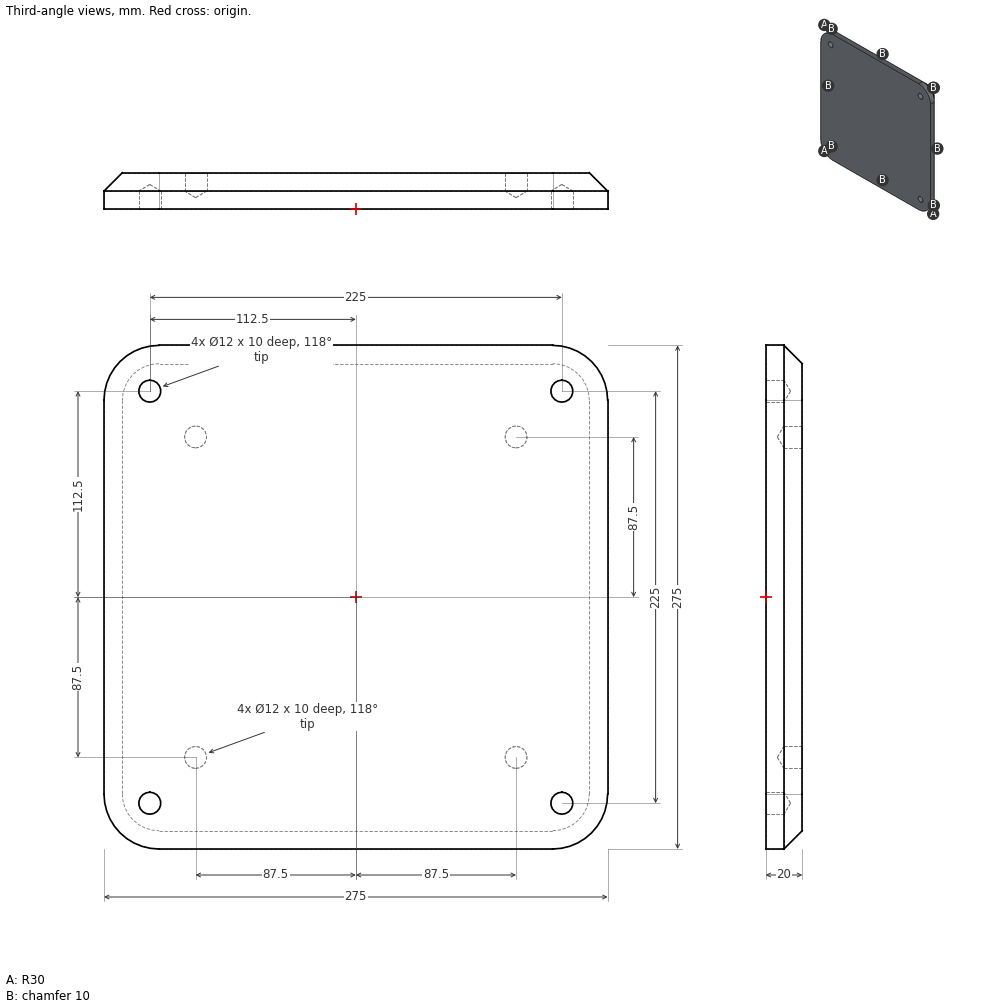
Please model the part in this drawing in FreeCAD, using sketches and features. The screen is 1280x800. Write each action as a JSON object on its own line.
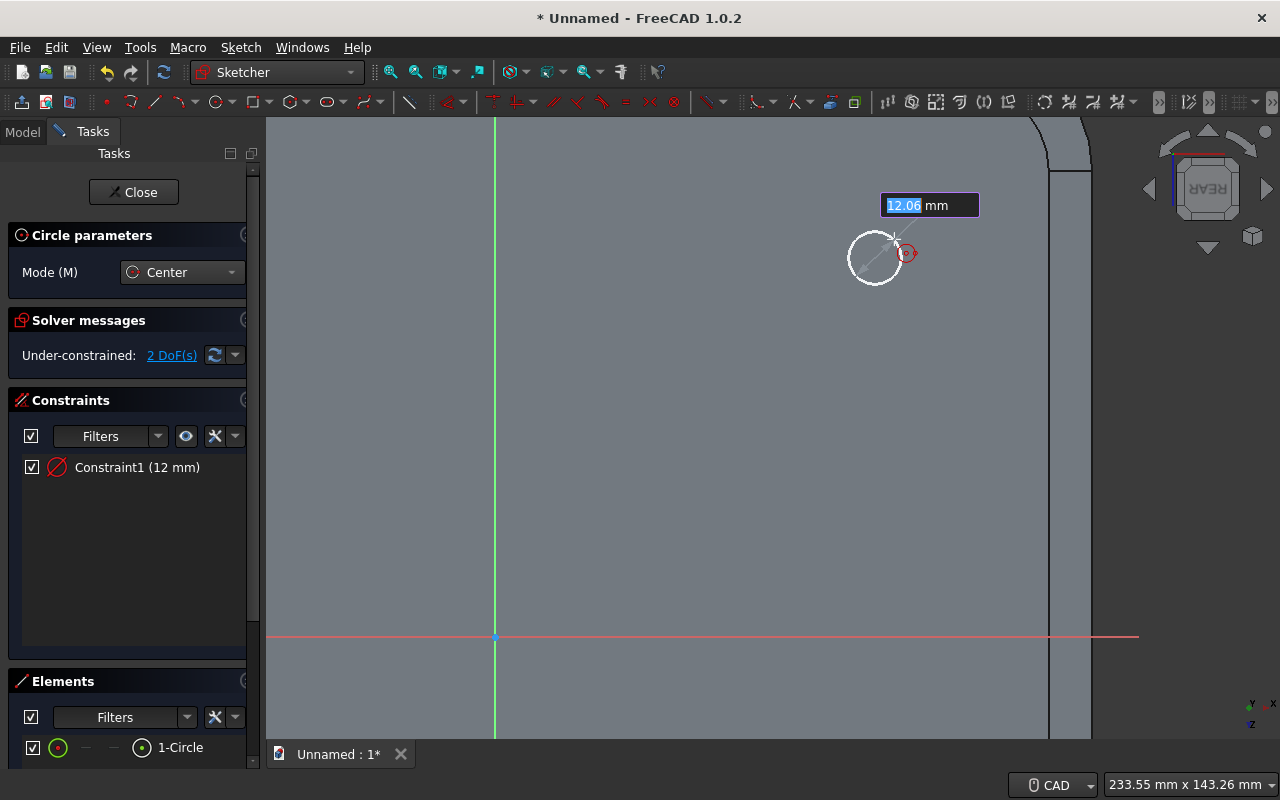
{"action": "type", "text": "12"}
{"action": "key", "text": "Return"}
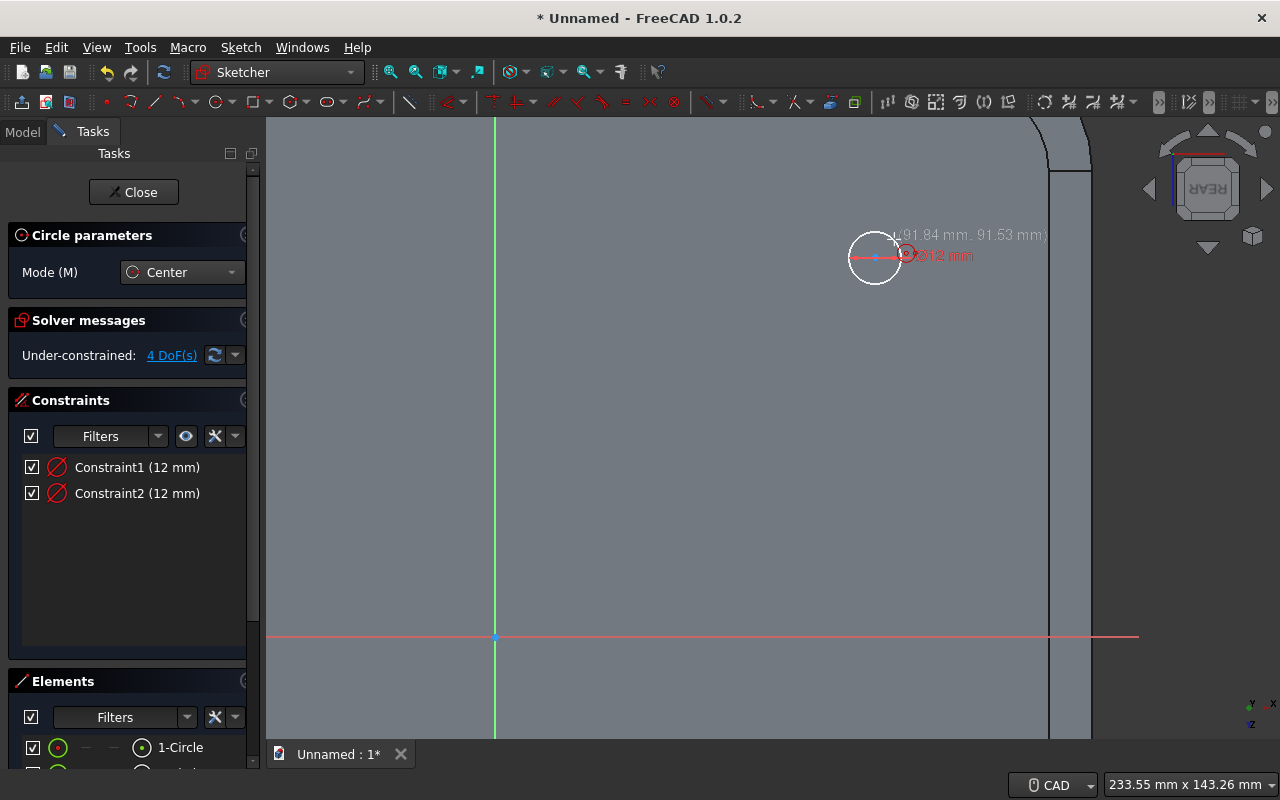
{"action": "scroll", "coordinate": [875, 257], "scroll_direction": "down", "scroll_amount": 4}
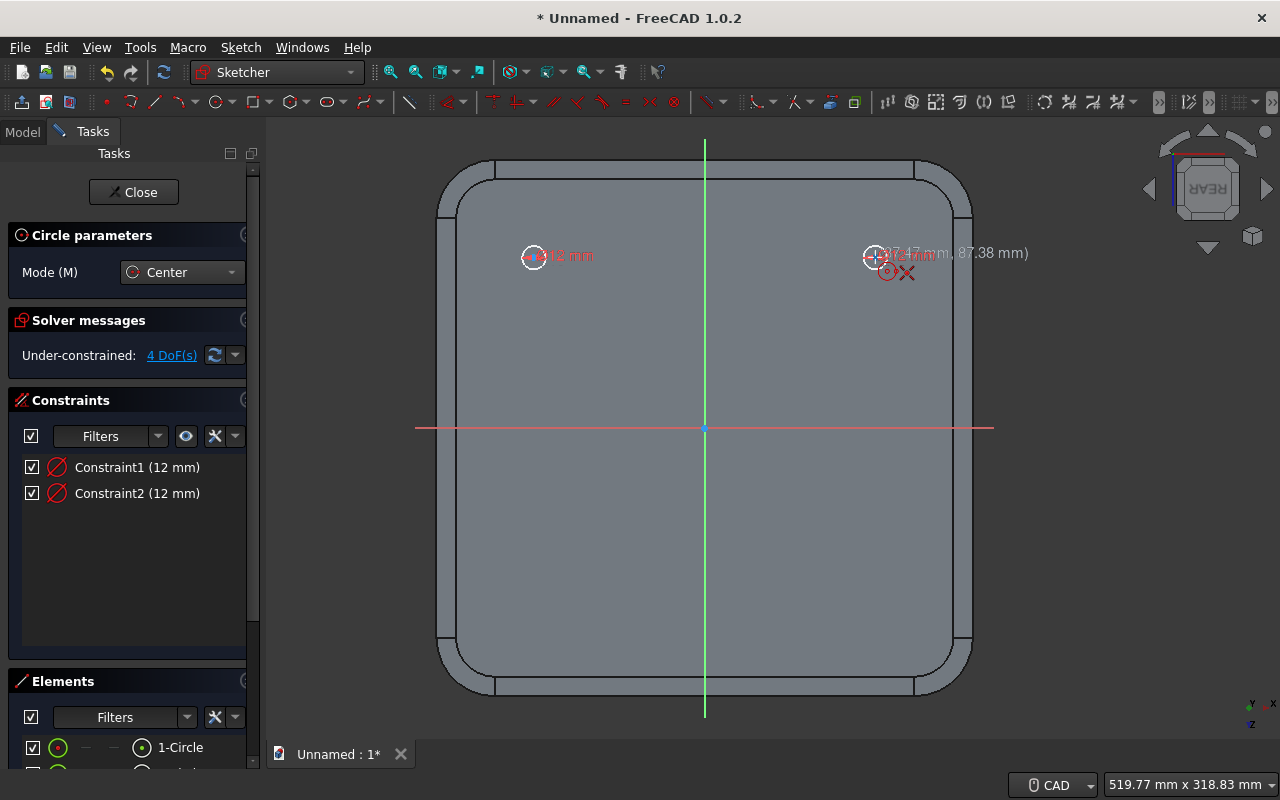
{"action": "scroll", "coordinate": [875, 599], "scroll_direction": "up", "scroll_amount": 4}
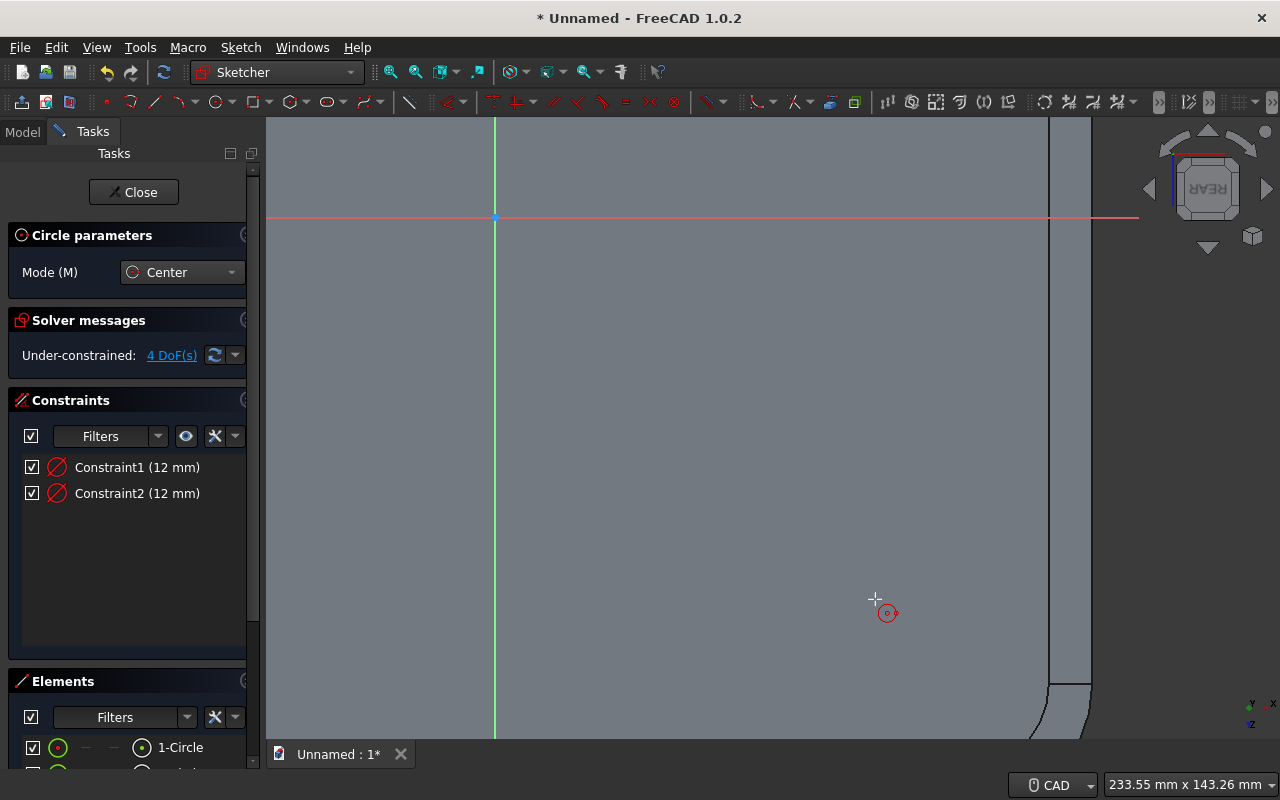
{"action": "left_click", "coordinate": [875, 597]}
{"action": "mouse_move", "coordinate": [894, 579]}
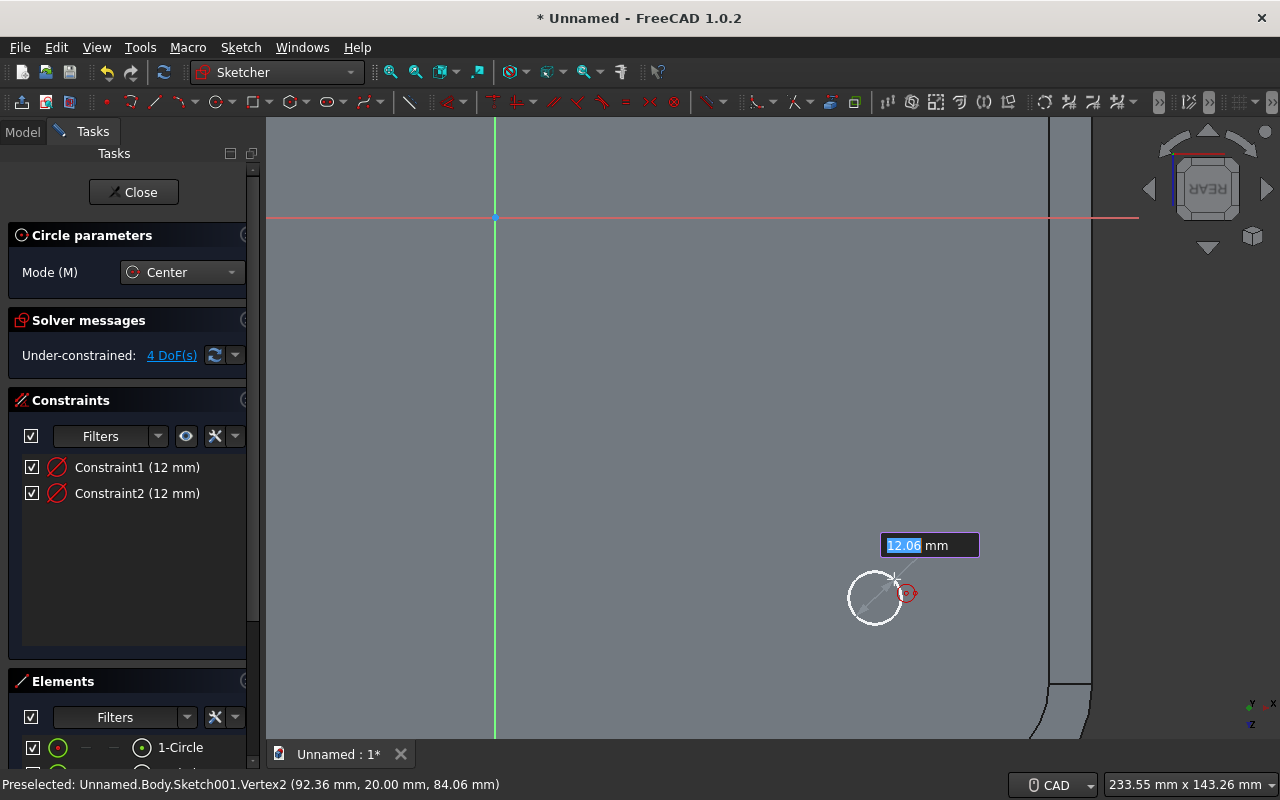
{"action": "type", "text": "12"}
{"action": "key", "text": "Return"}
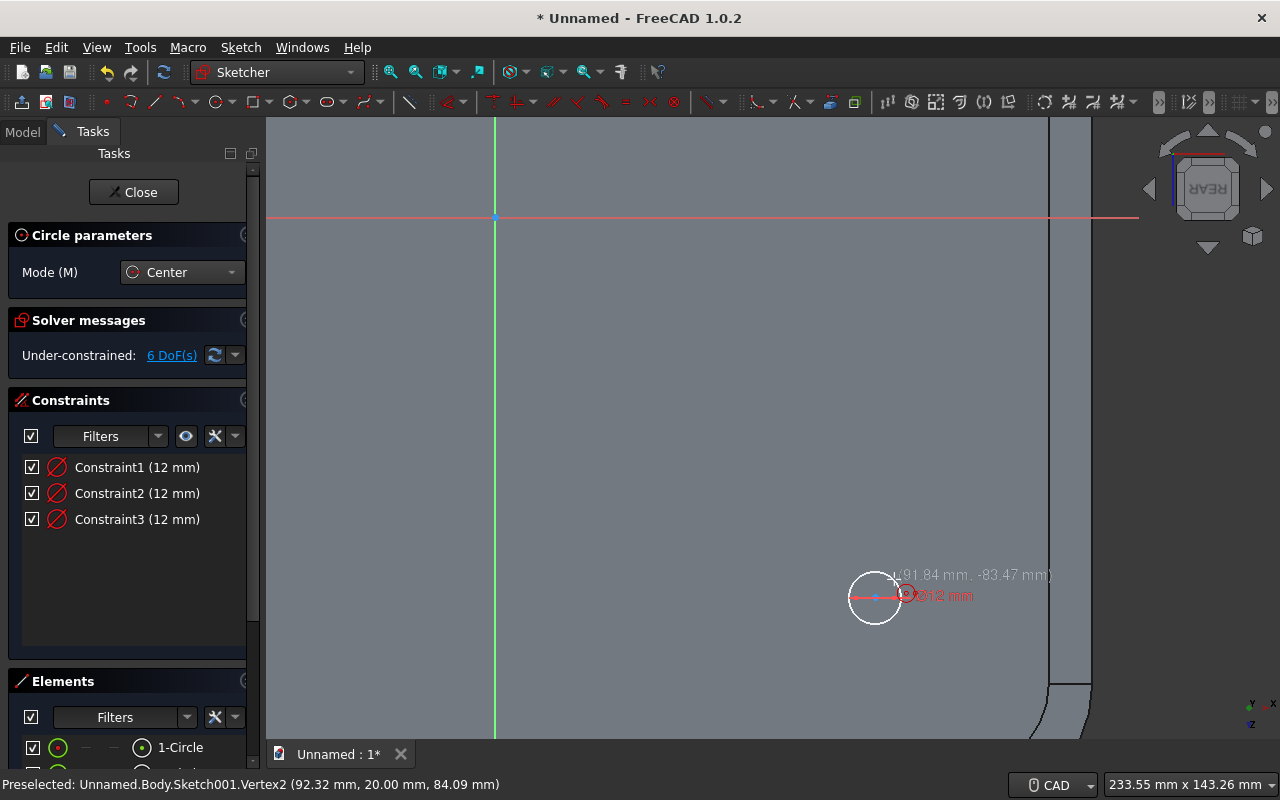
{"action": "scroll", "coordinate": [875, 600], "scroll_direction": "down", "scroll_amount": 4}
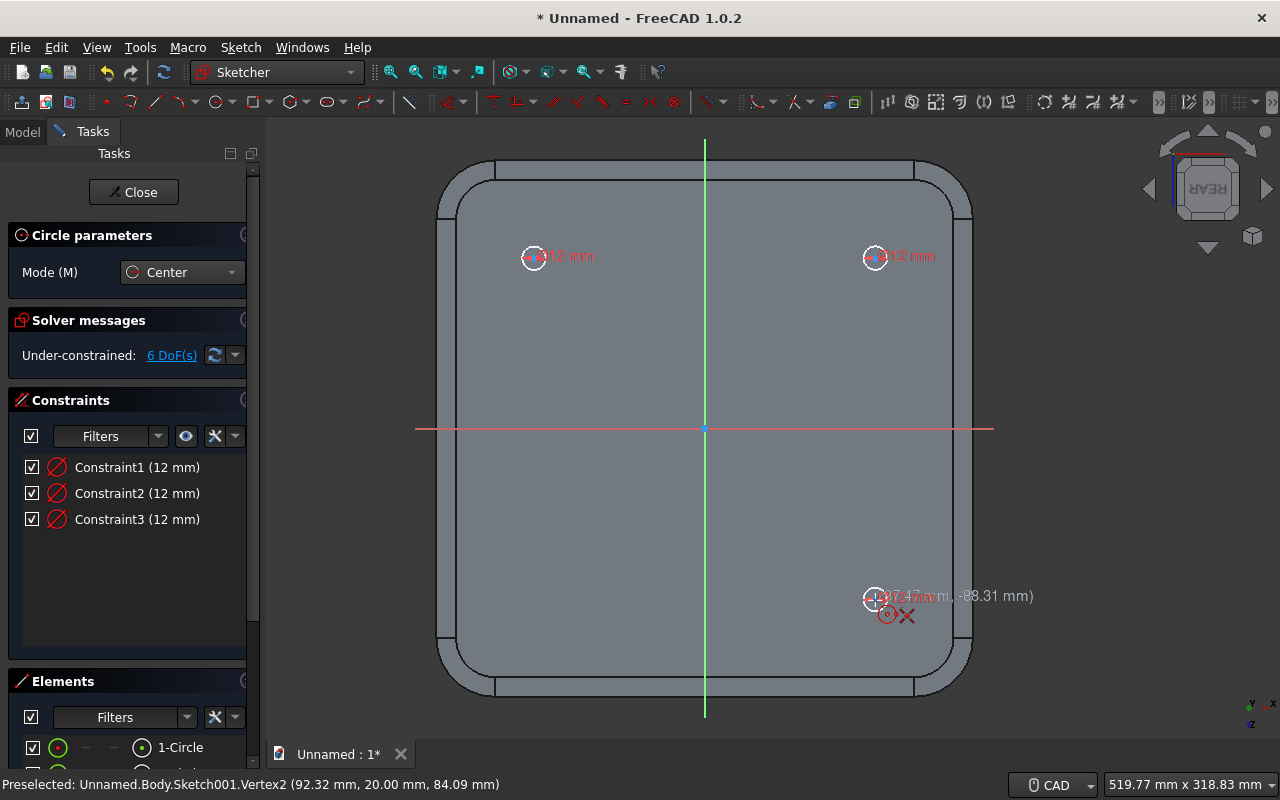
{"action": "scroll", "coordinate": [534, 599], "scroll_direction": "up", "scroll_amount": 4}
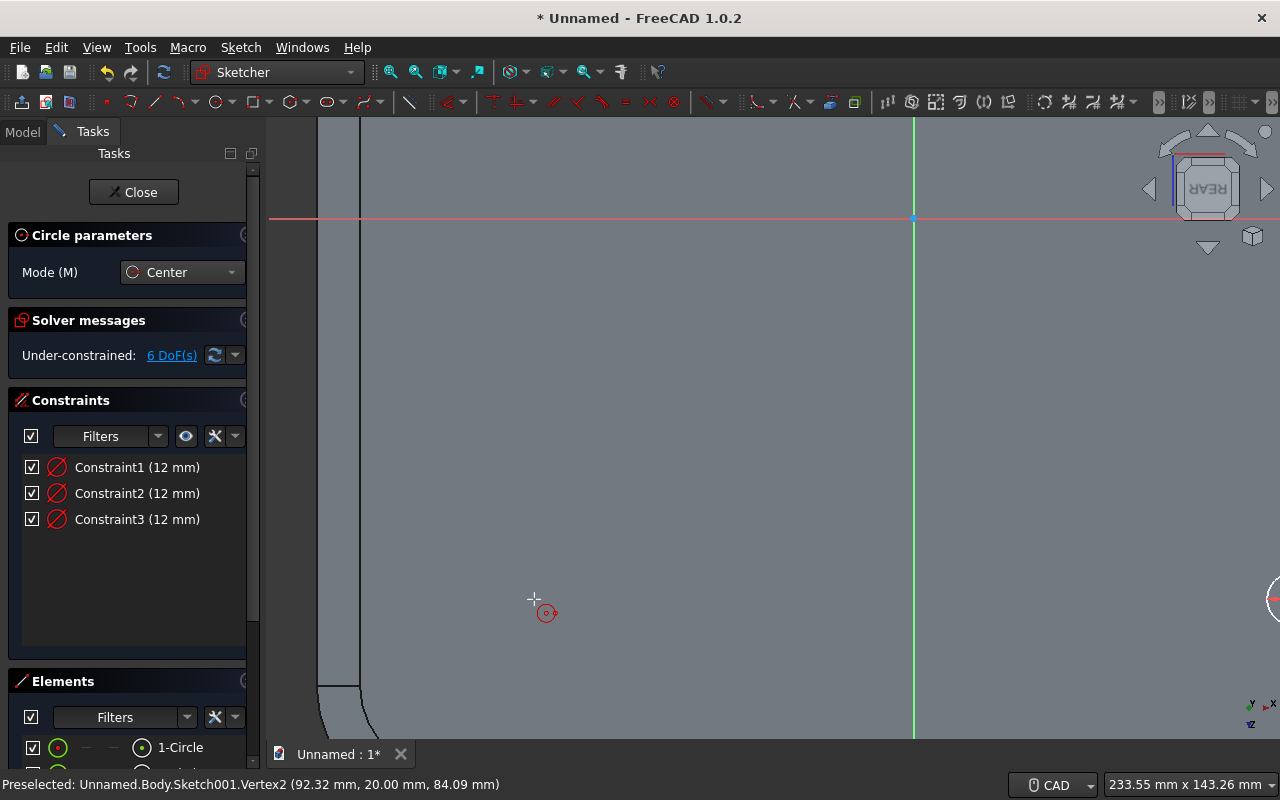
{"action": "left_click", "coordinate": [534, 599]}
{"action": "mouse_move", "coordinate": [552, 580]}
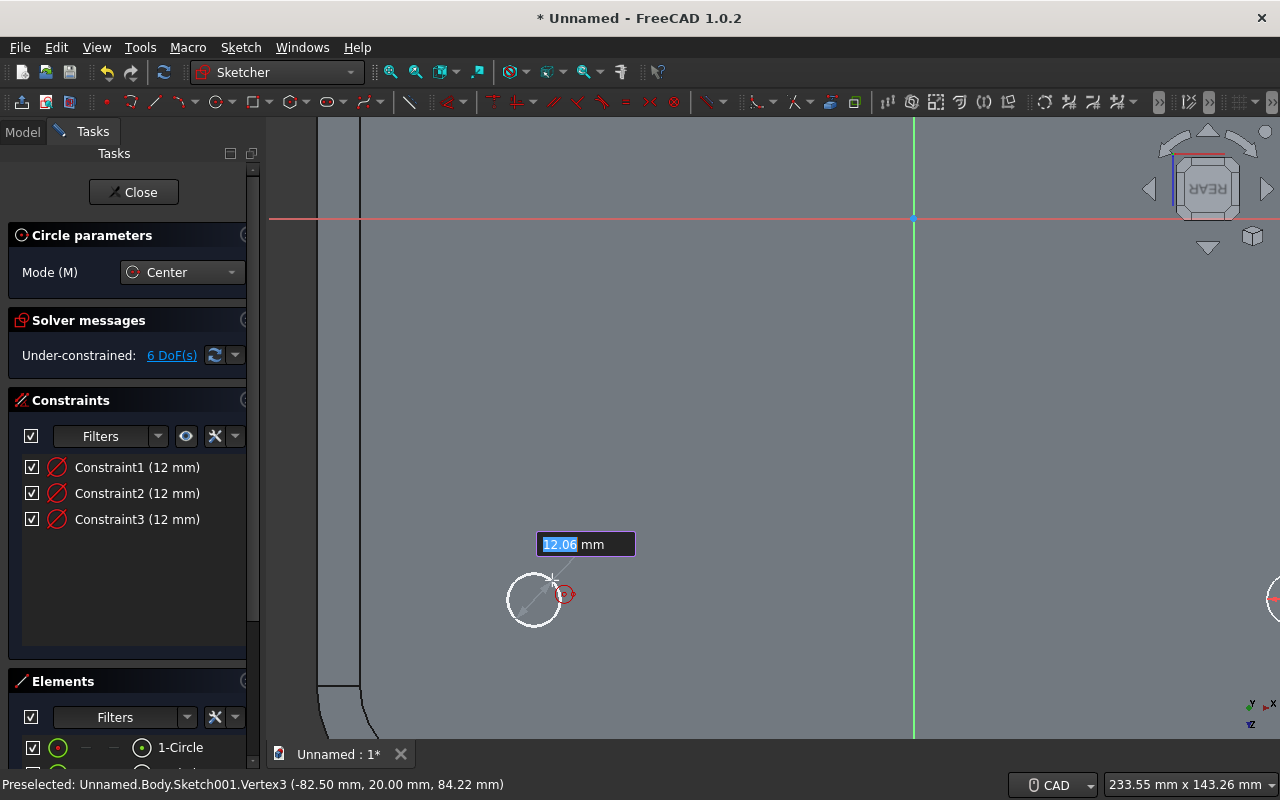
{"action": "type", "text": "12"}
{"action": "key", "text": "Return"}
{"action": "key", "text": "Escape"}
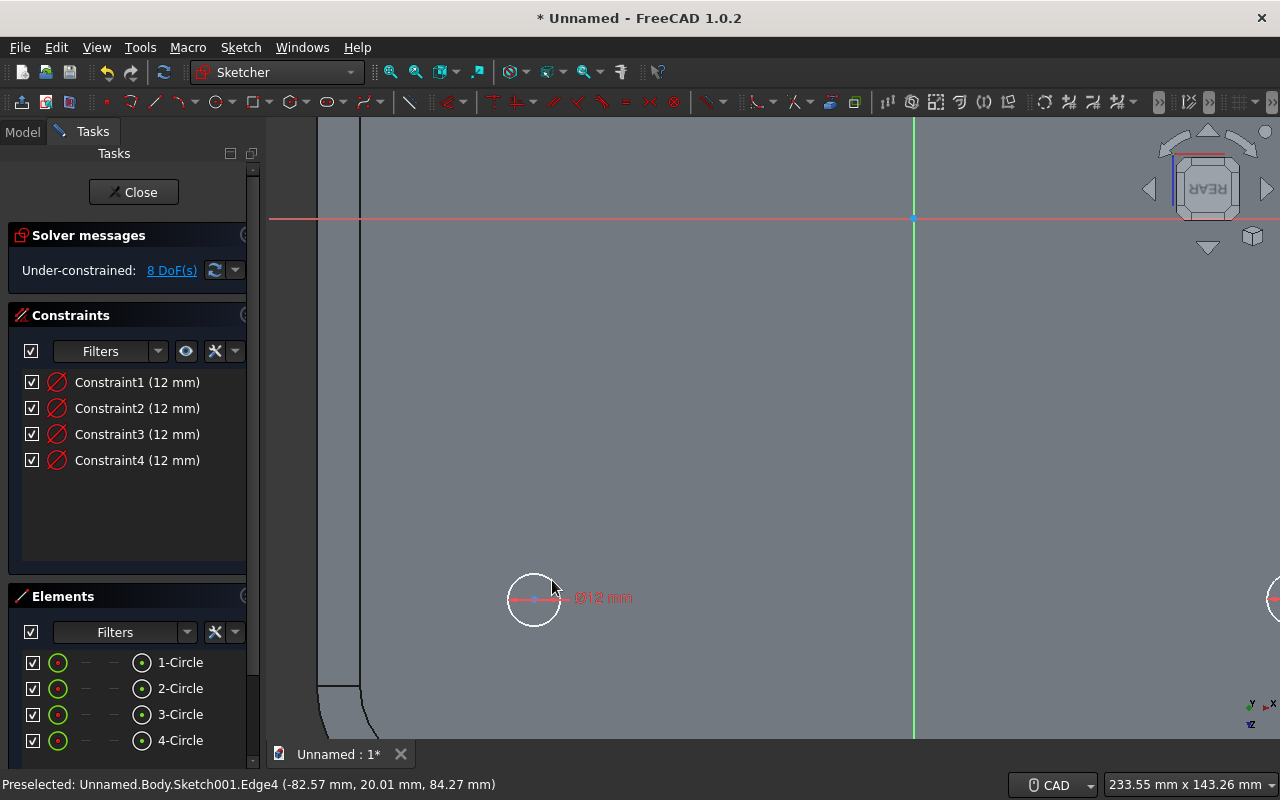
{"action": "scroll", "coordinate": [534, 599], "scroll_direction": "down", "scroll_amount": 4}